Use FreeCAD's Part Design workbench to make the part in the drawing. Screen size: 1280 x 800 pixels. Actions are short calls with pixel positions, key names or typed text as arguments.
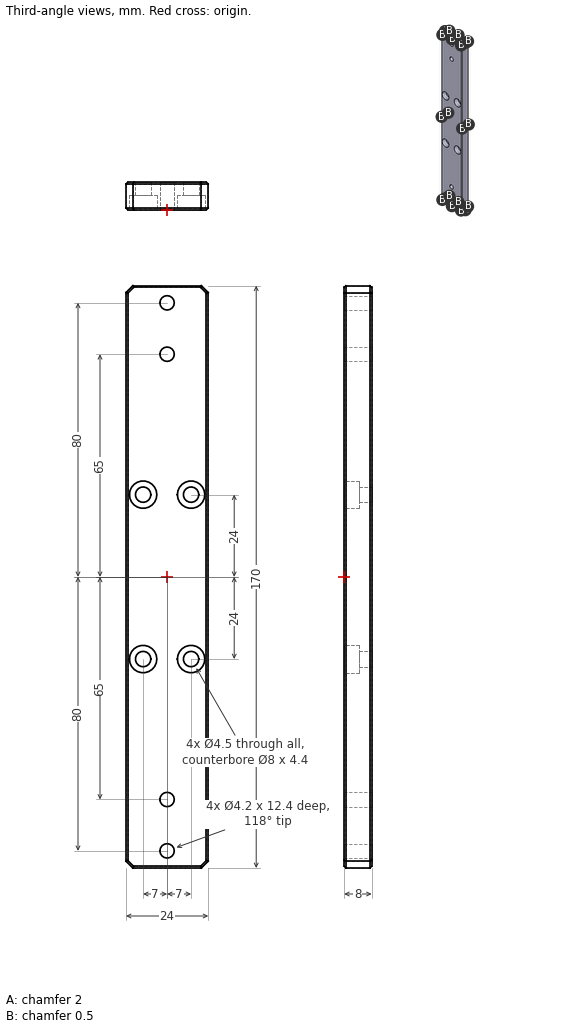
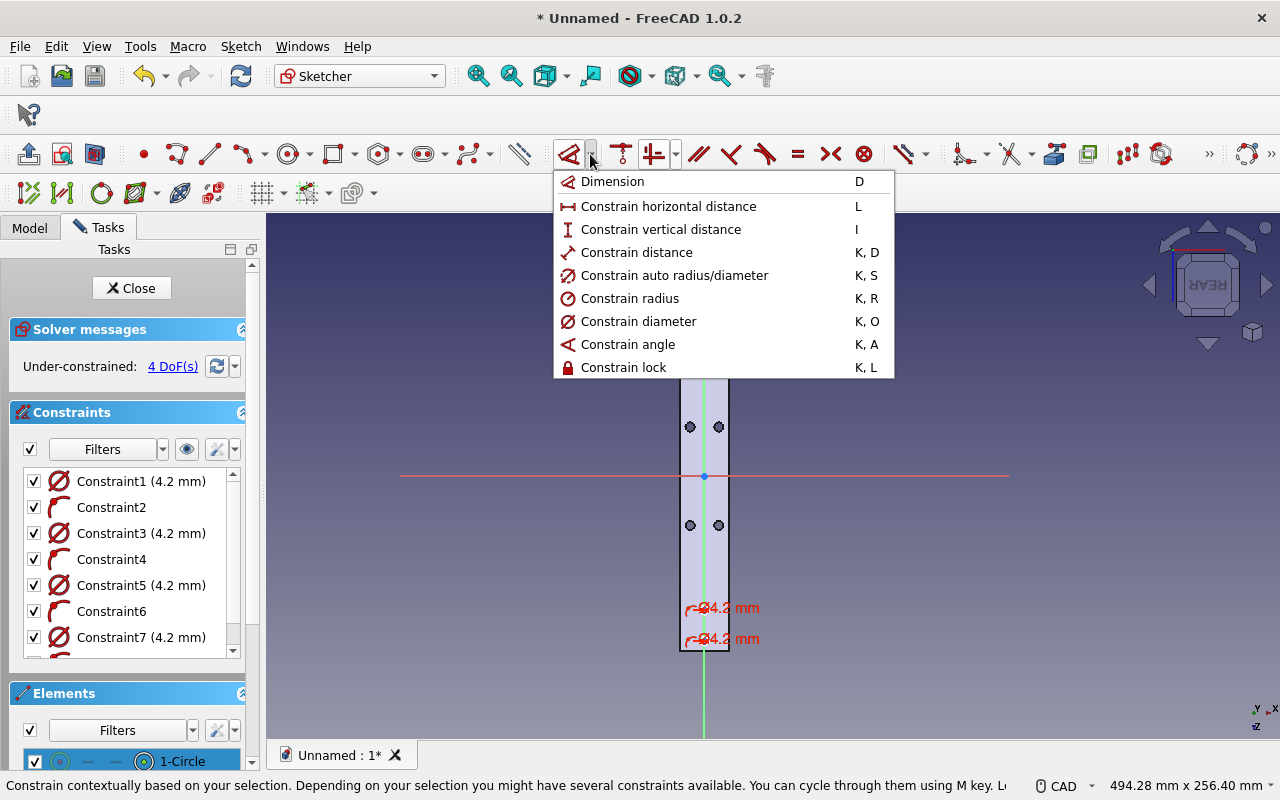
click(724, 230)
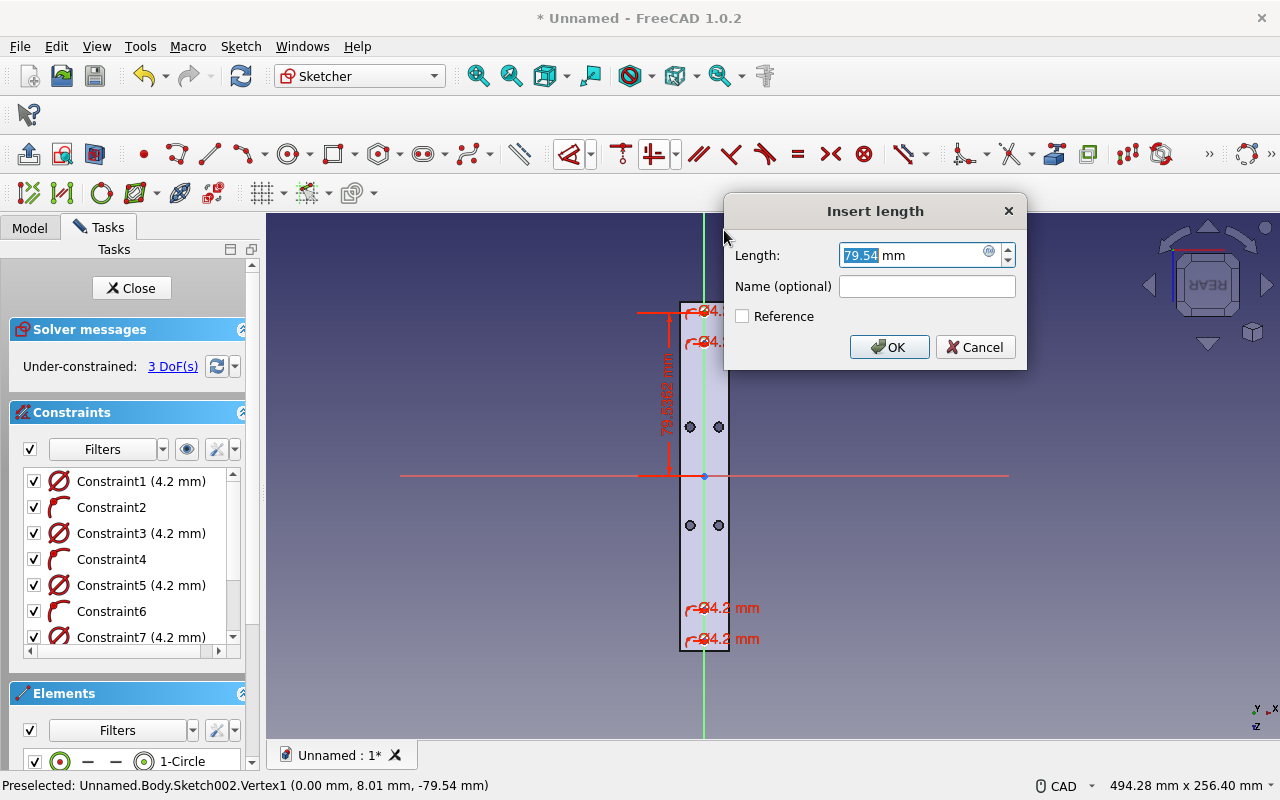
text(80)
key(Return)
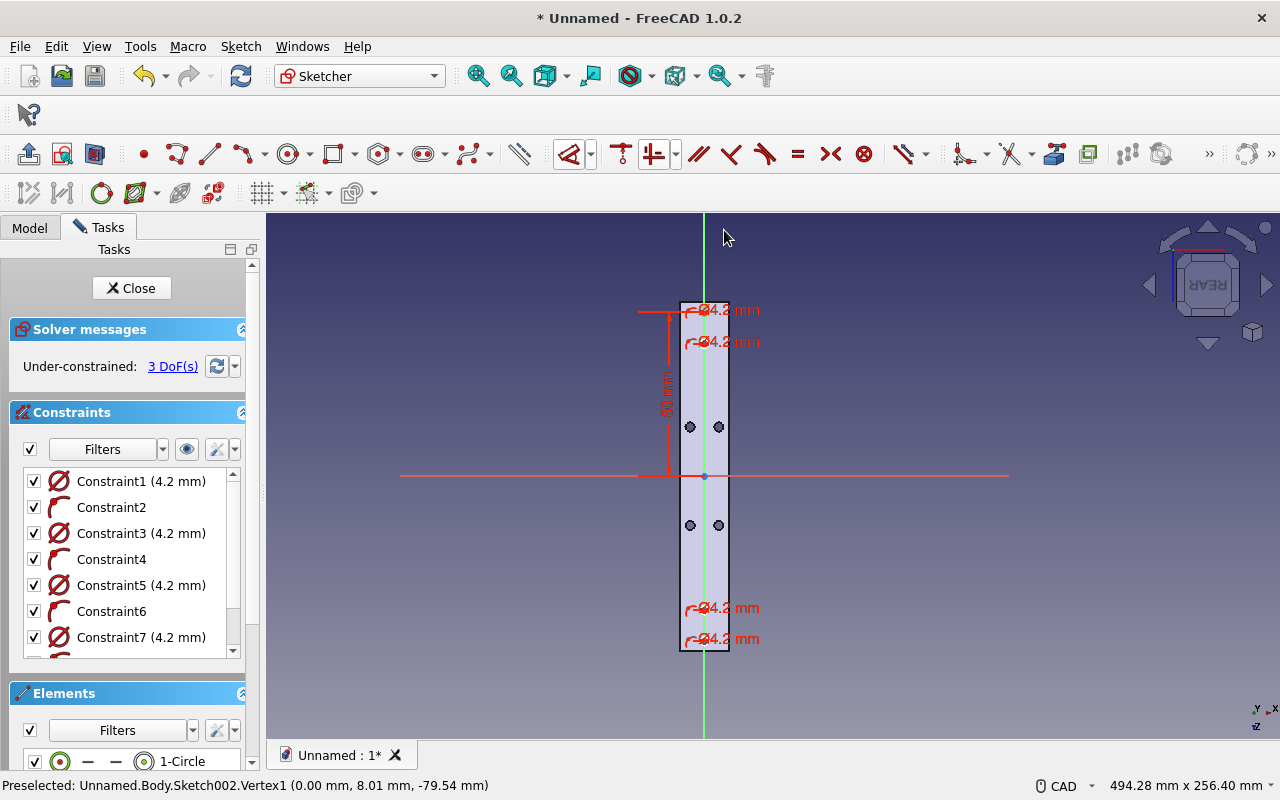
click(704, 641)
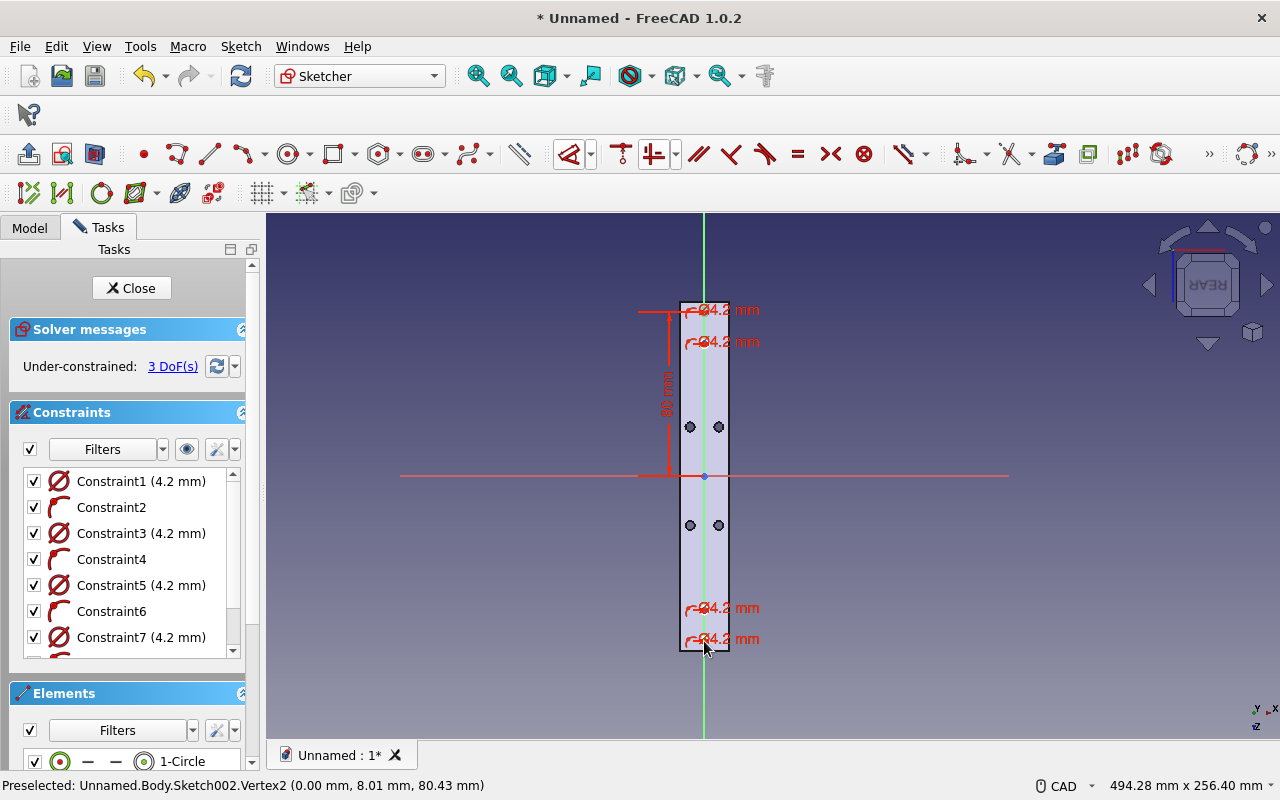
click(590, 154)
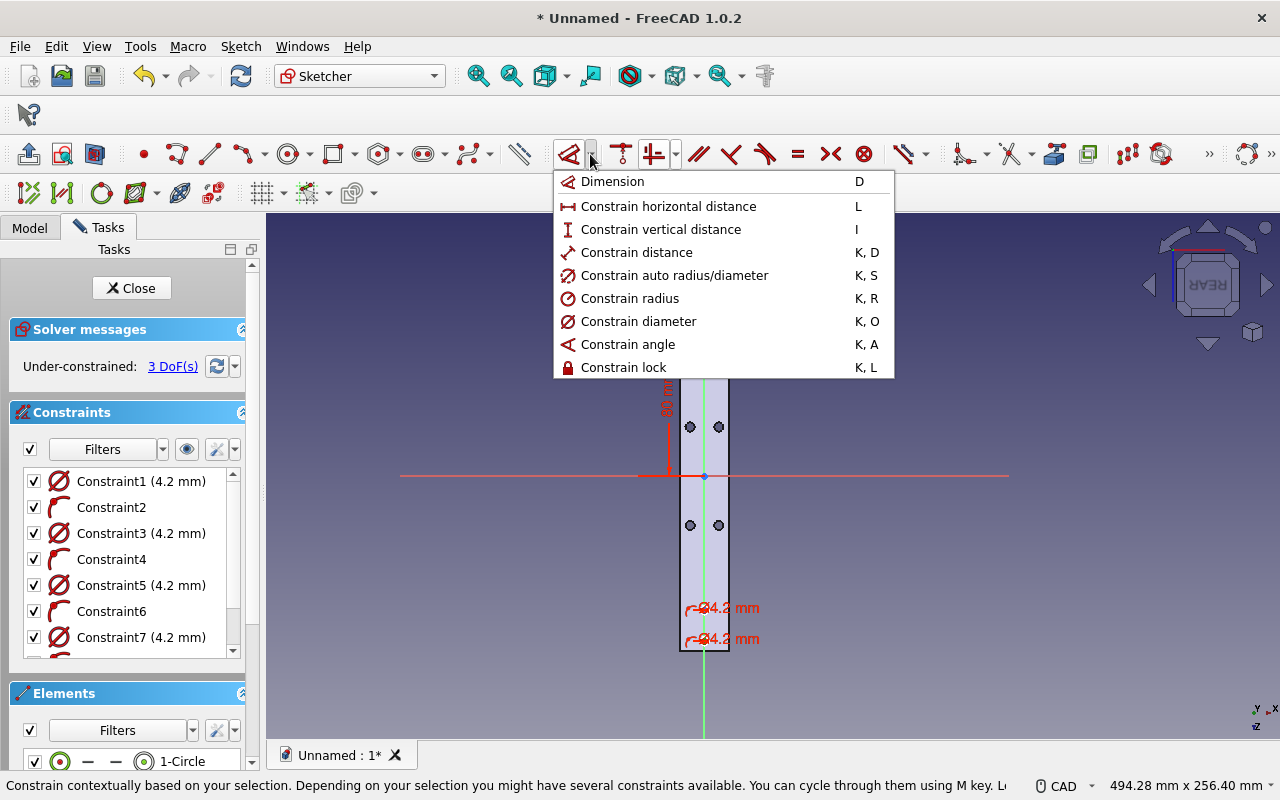
click(724, 230)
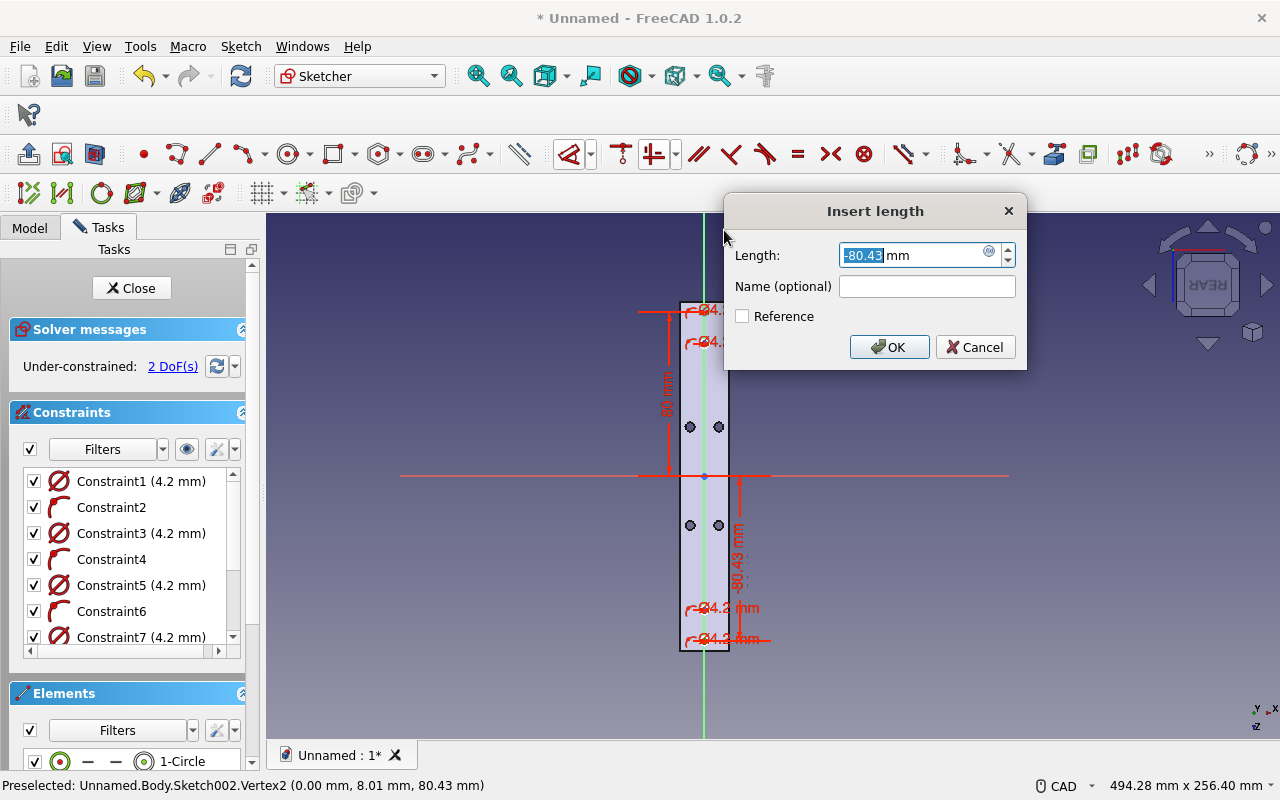
text(-80)
key(Return)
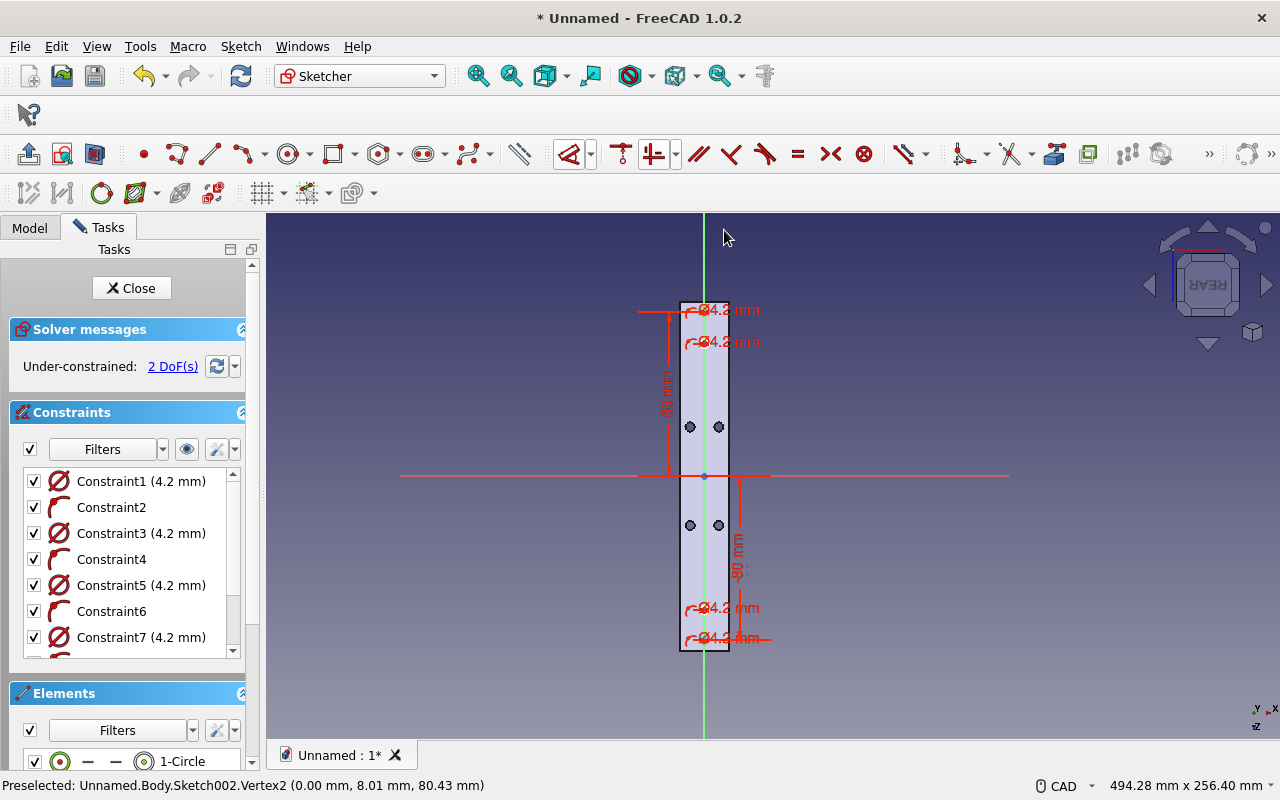
click(704, 610)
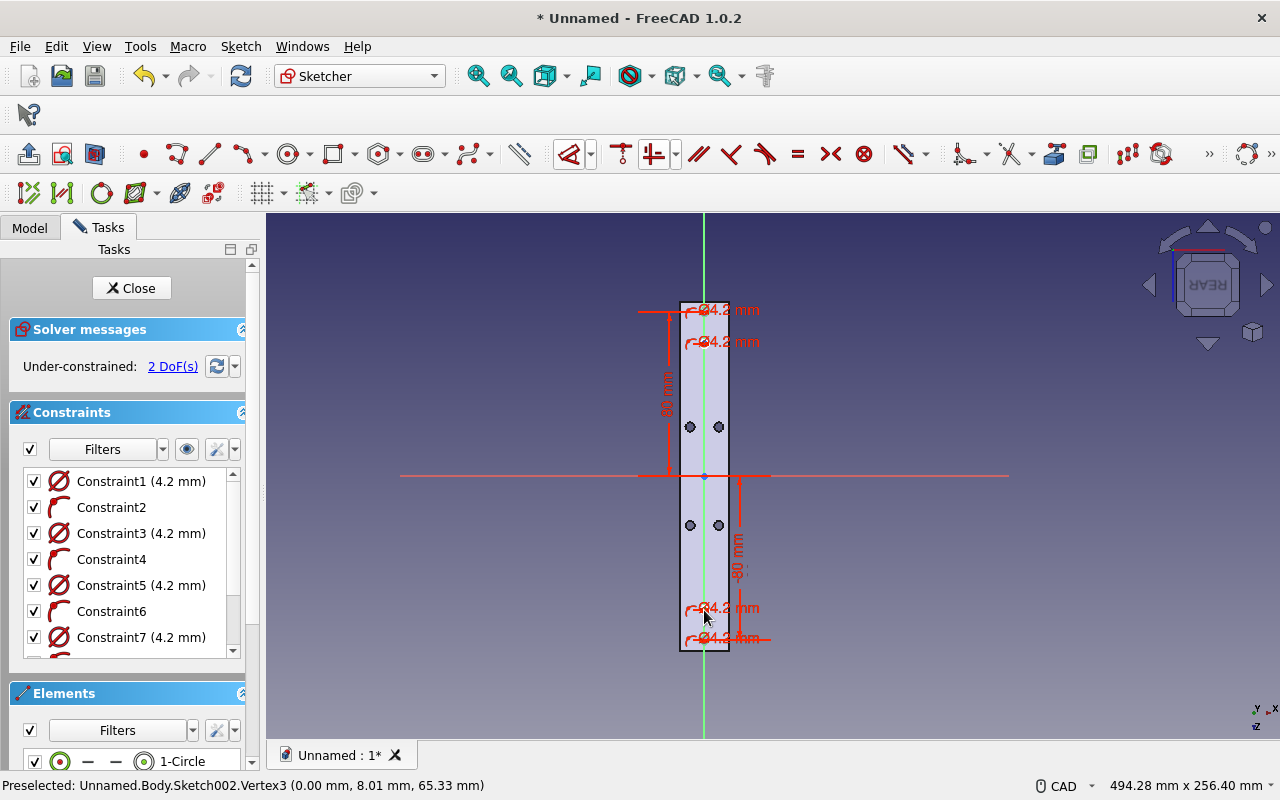
key(i)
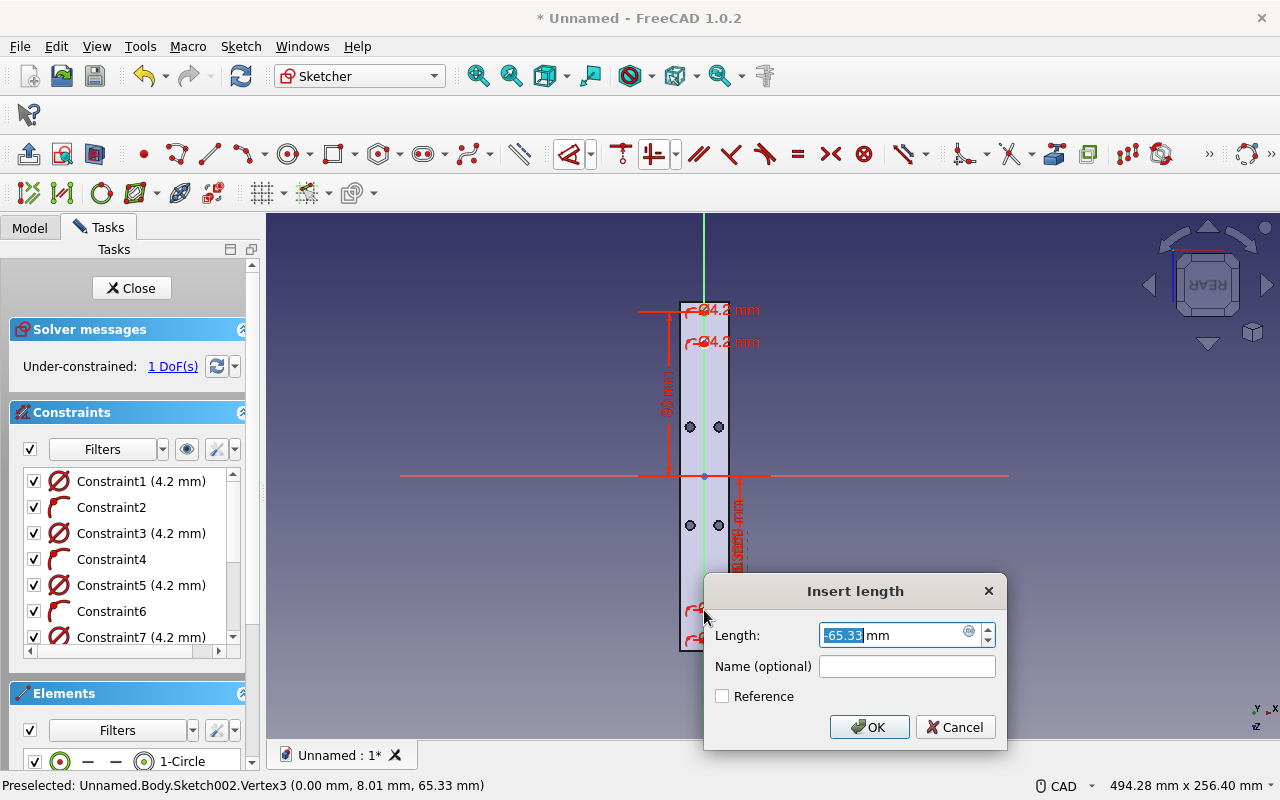
text(-65)
key(Return)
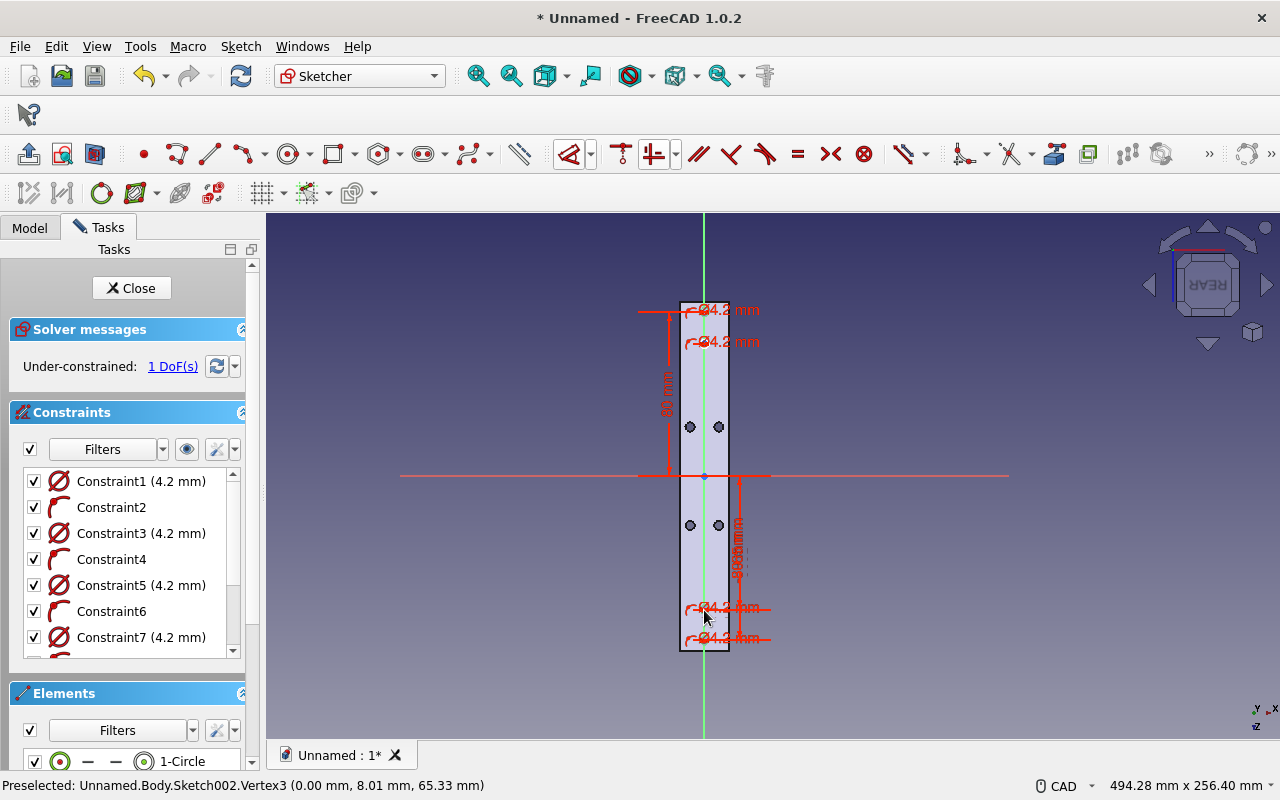
click(704, 344)